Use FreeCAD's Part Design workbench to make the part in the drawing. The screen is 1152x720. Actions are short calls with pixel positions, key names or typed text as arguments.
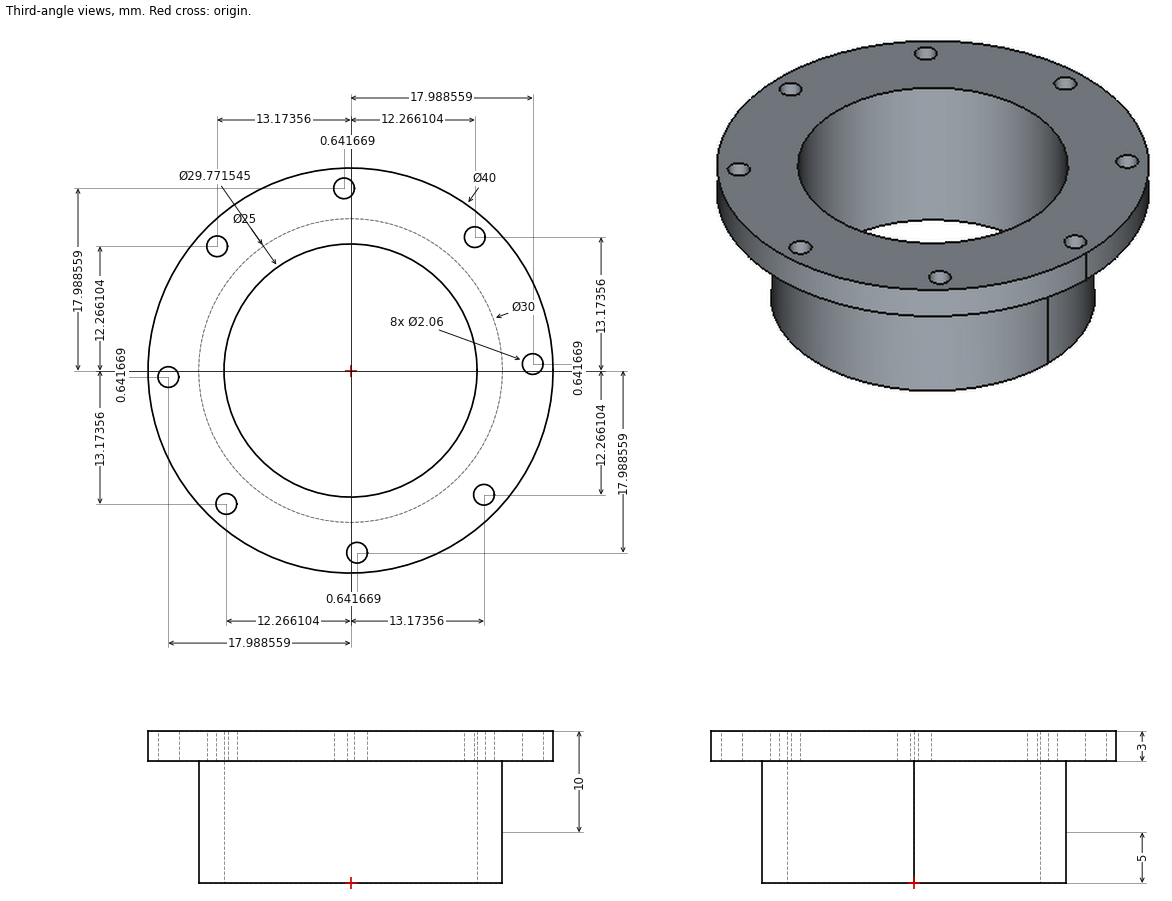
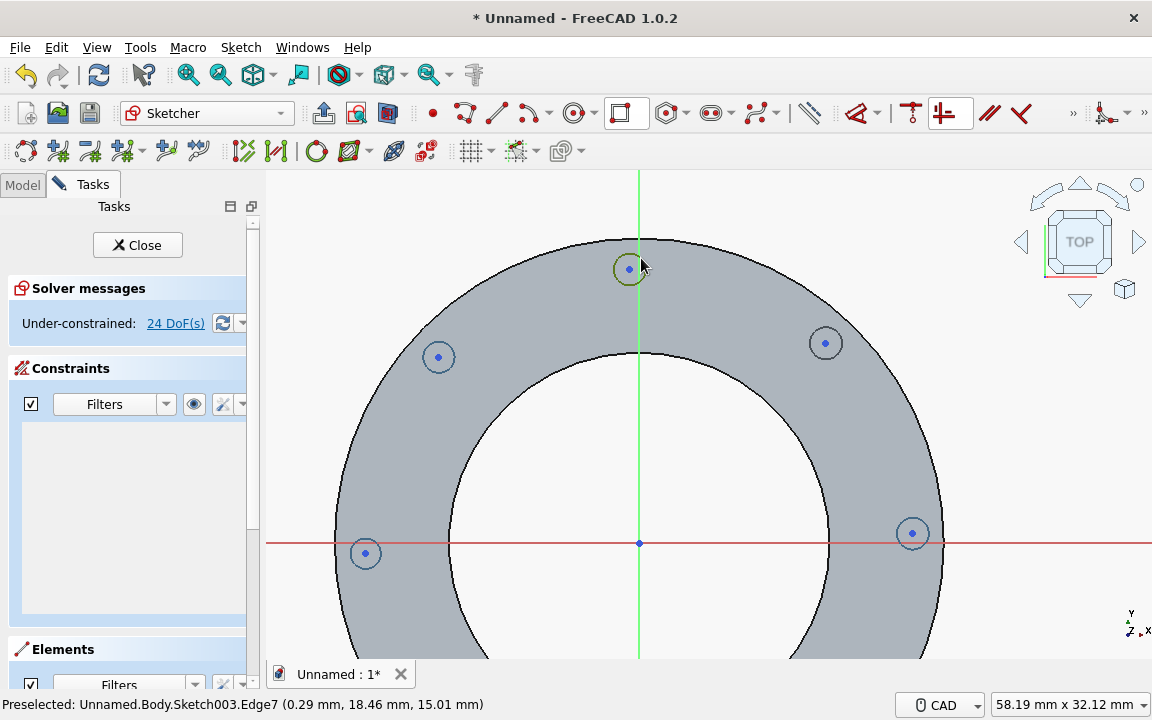
click(837, 332)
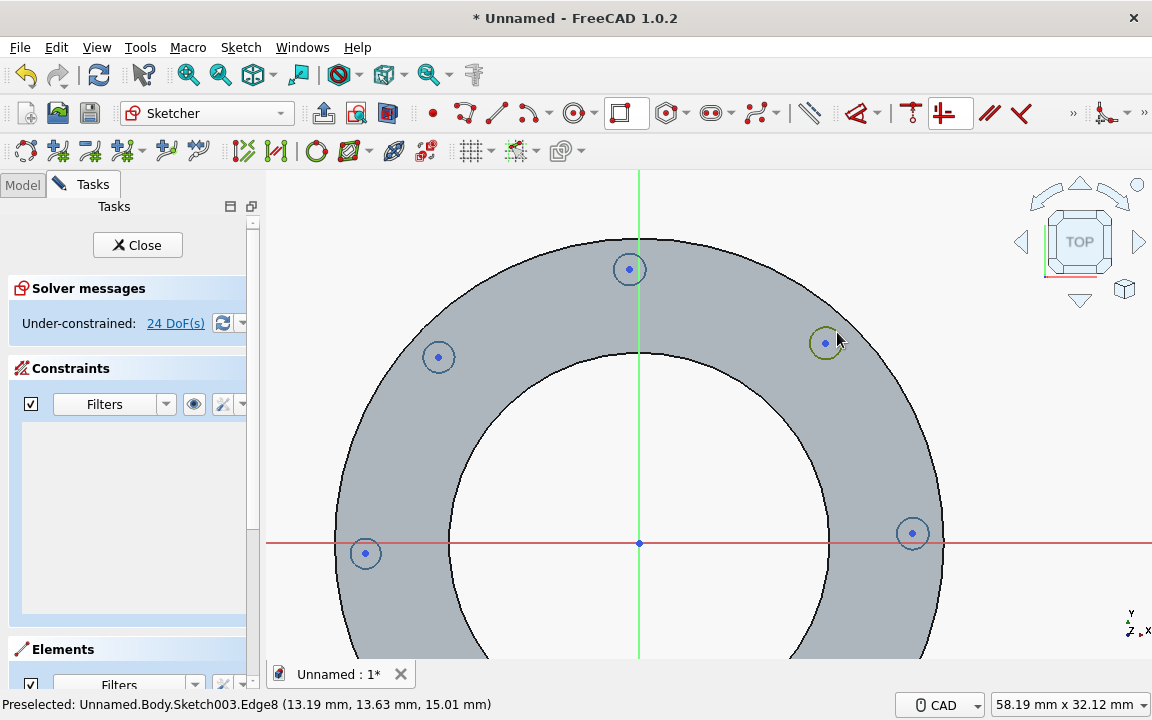
key(e)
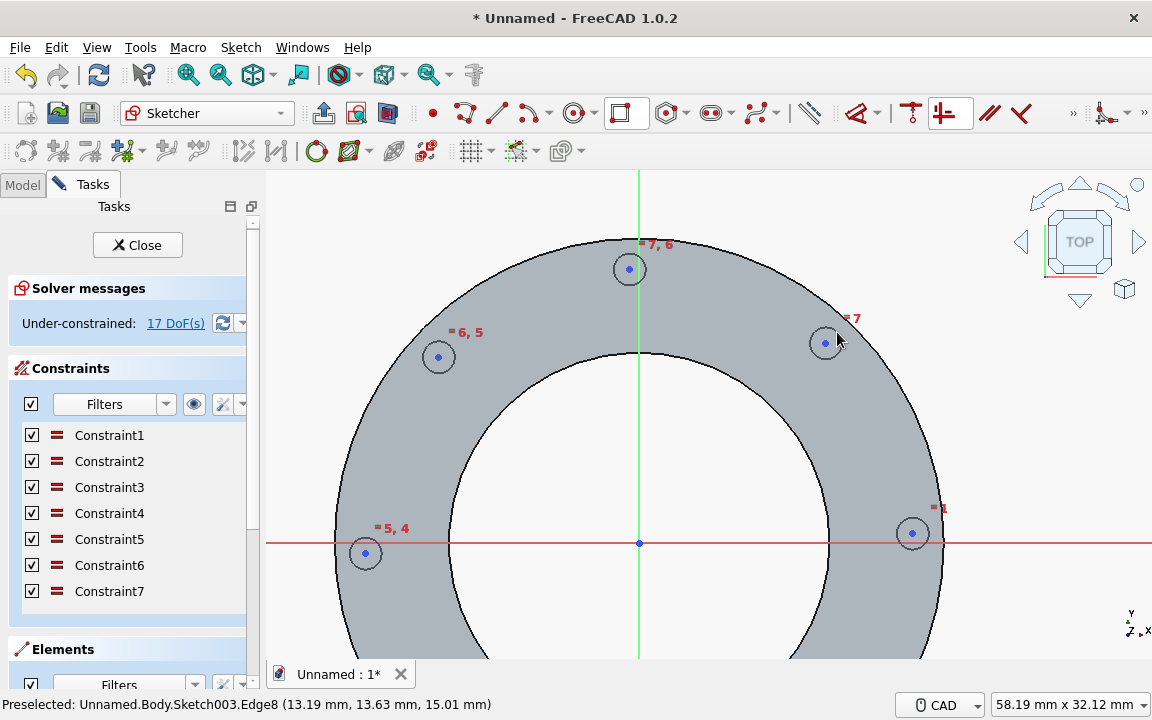
key(d)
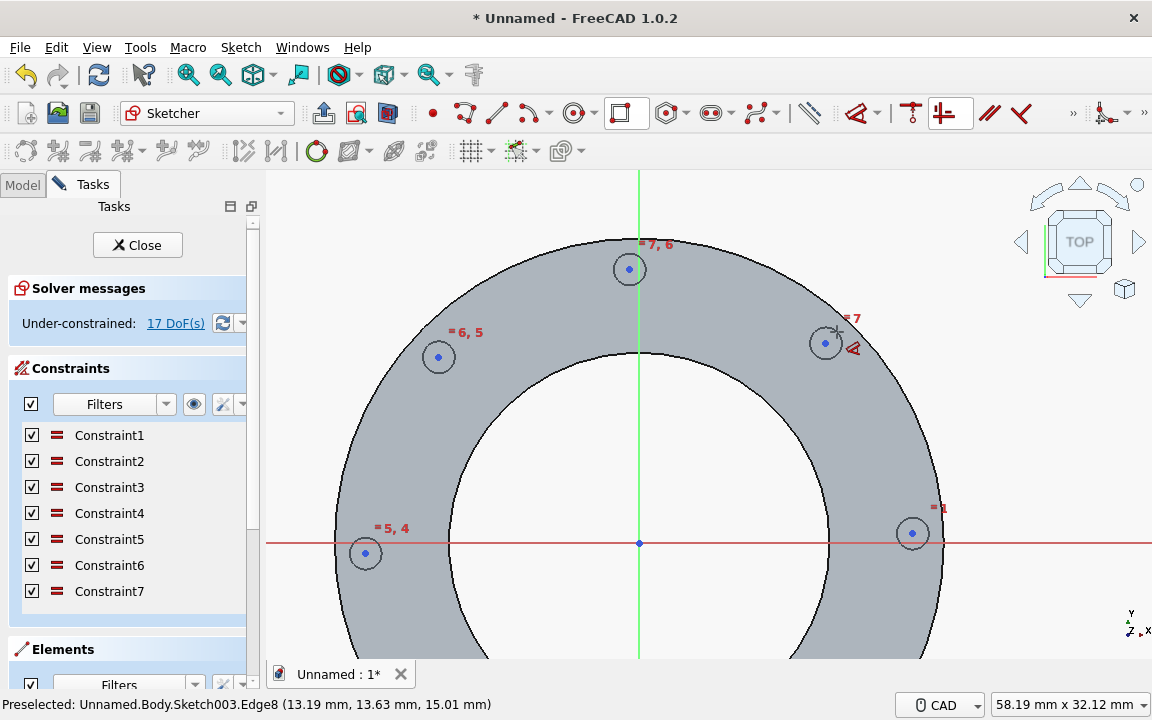
scroll(924, 522, up, 2)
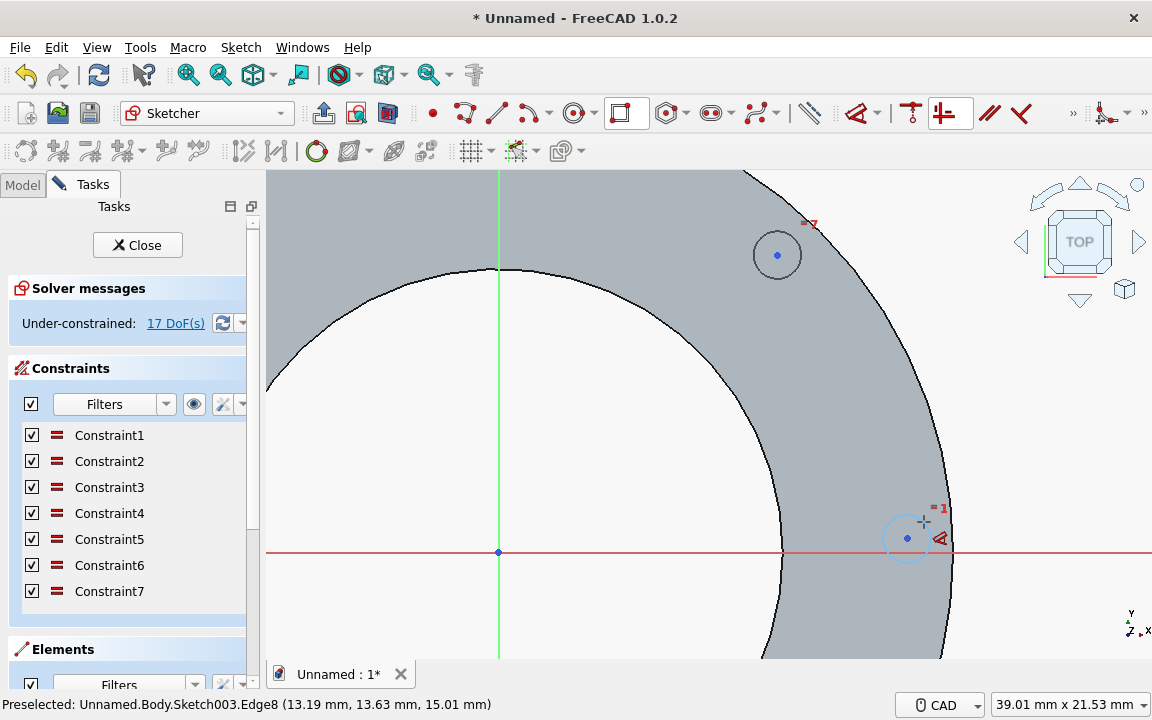
click(924, 522)
click(947, 499)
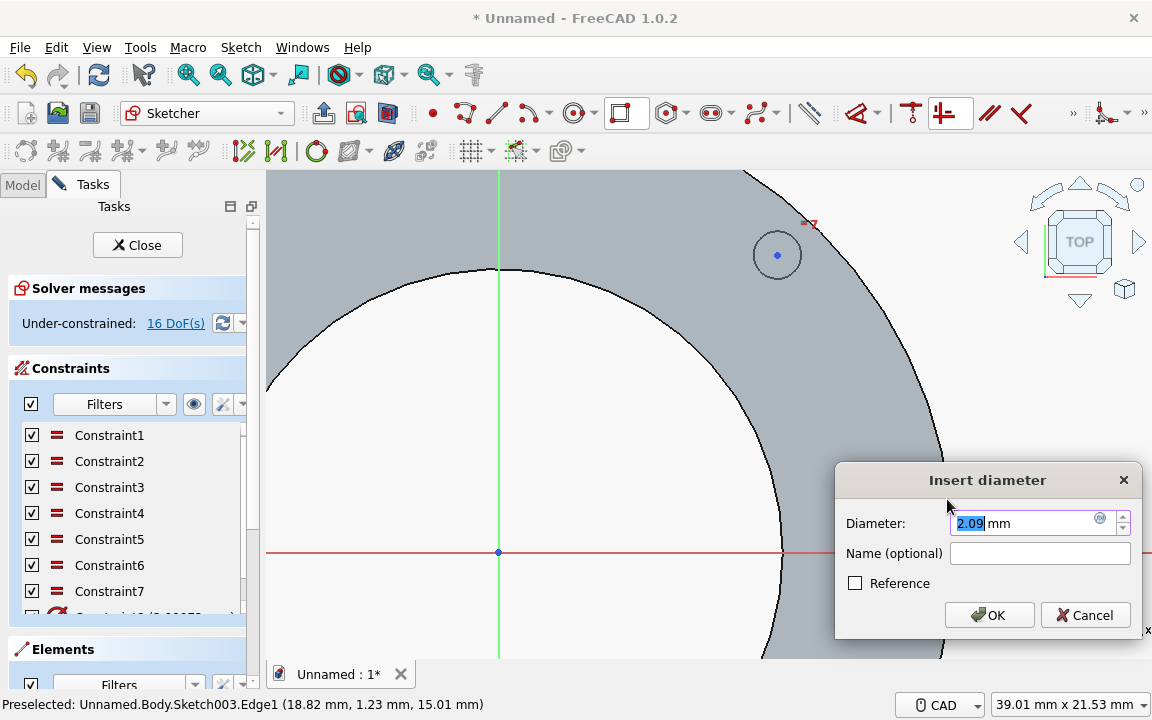
text(2.06)
key(Return)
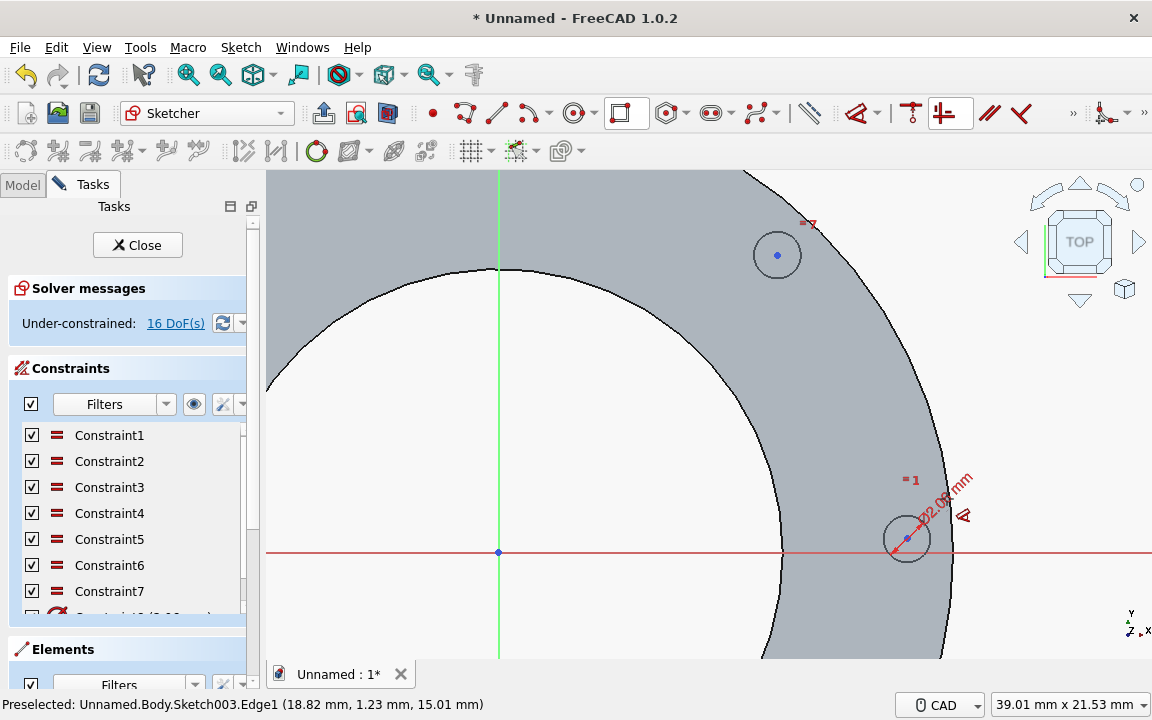
scroll(907, 539, up, 6)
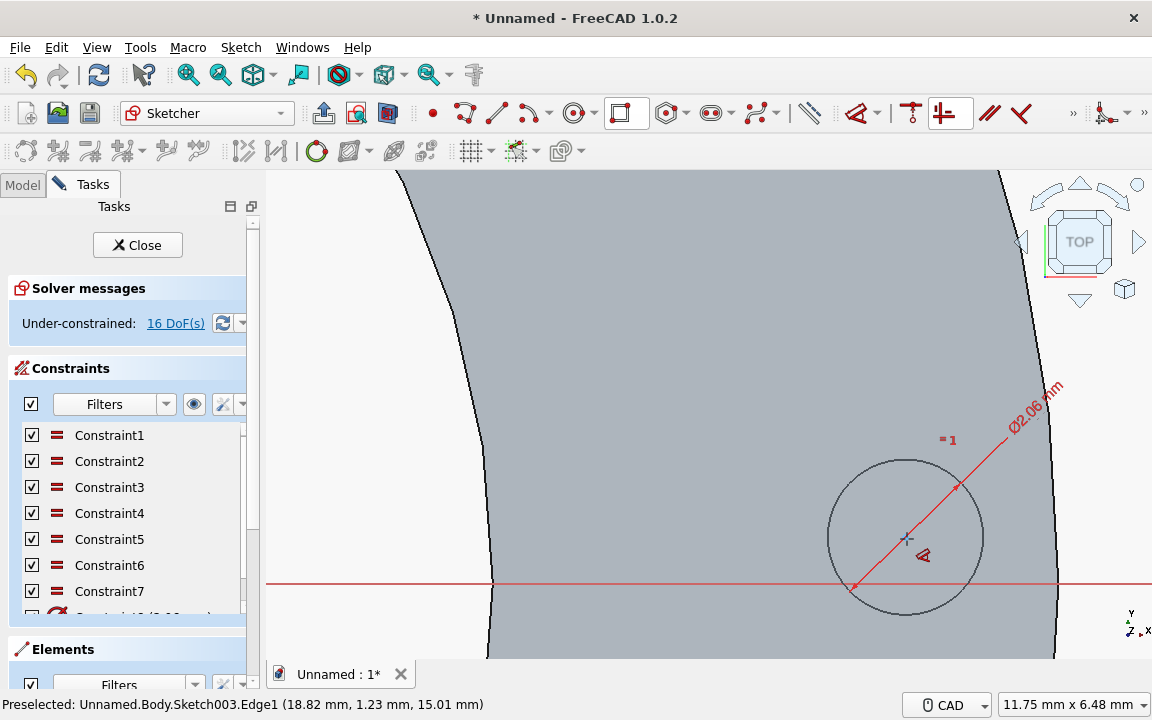
click(905, 537)
click(939, 560)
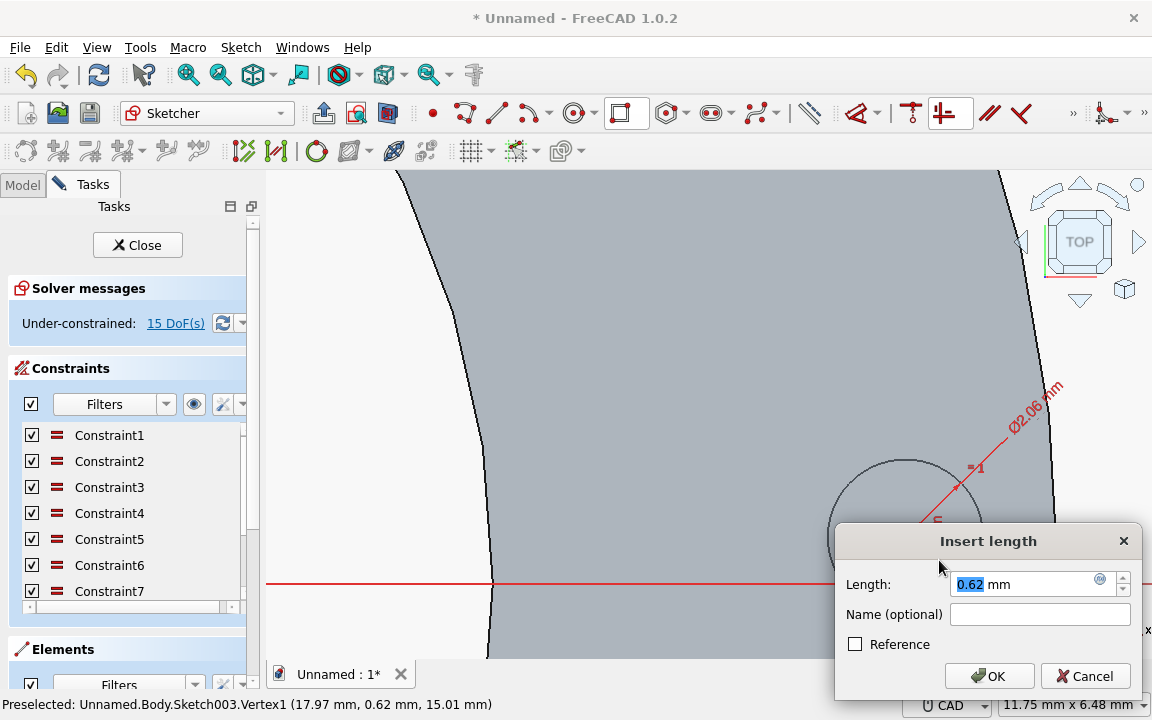
text(0.641669)
key(Return)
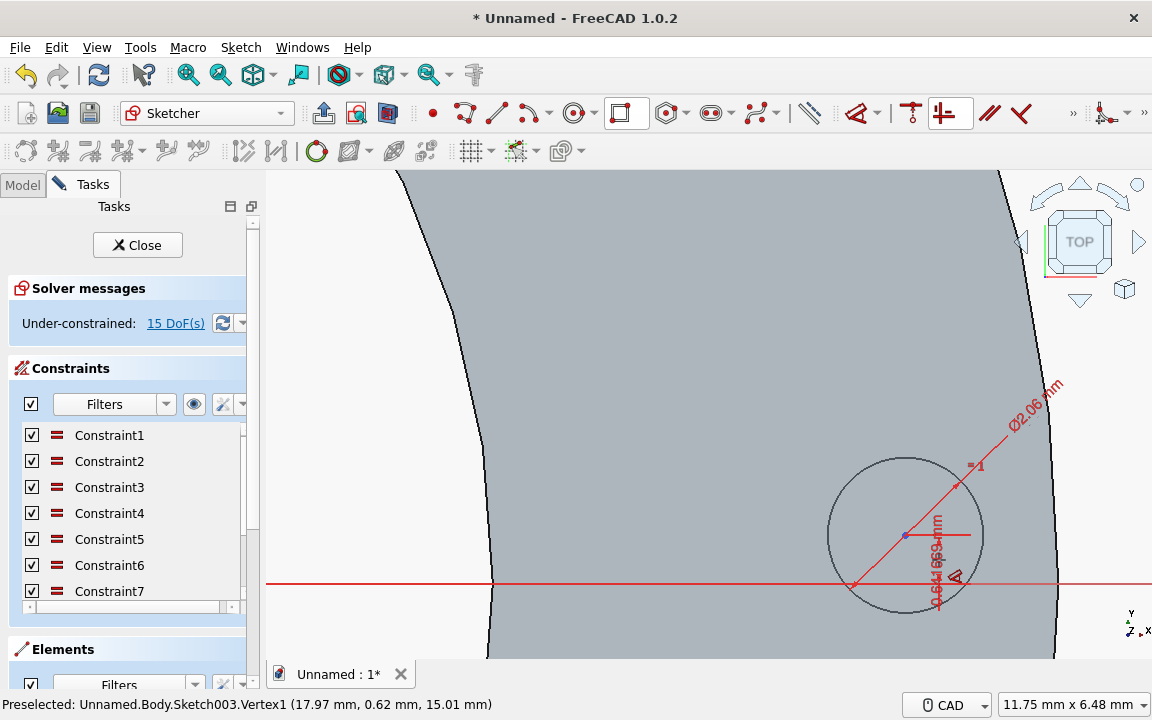
scroll(776, 393, down, 11)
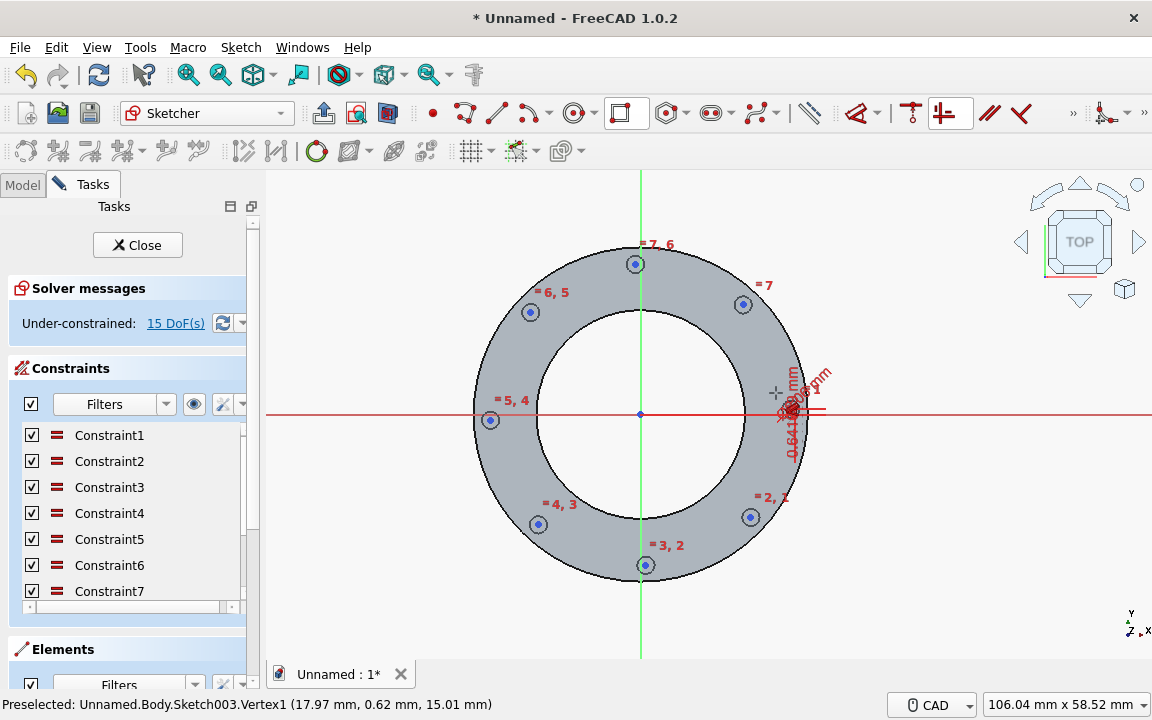
click(751, 517)
click(696, 551)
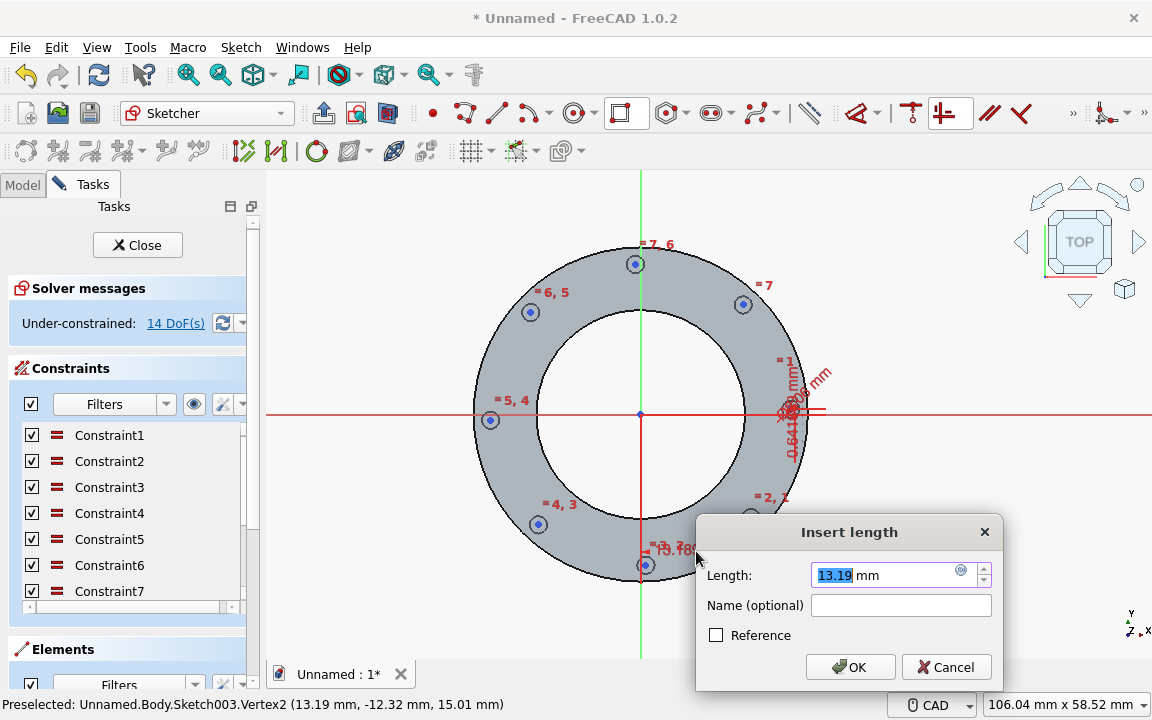
text(13.17356)
key(Return)